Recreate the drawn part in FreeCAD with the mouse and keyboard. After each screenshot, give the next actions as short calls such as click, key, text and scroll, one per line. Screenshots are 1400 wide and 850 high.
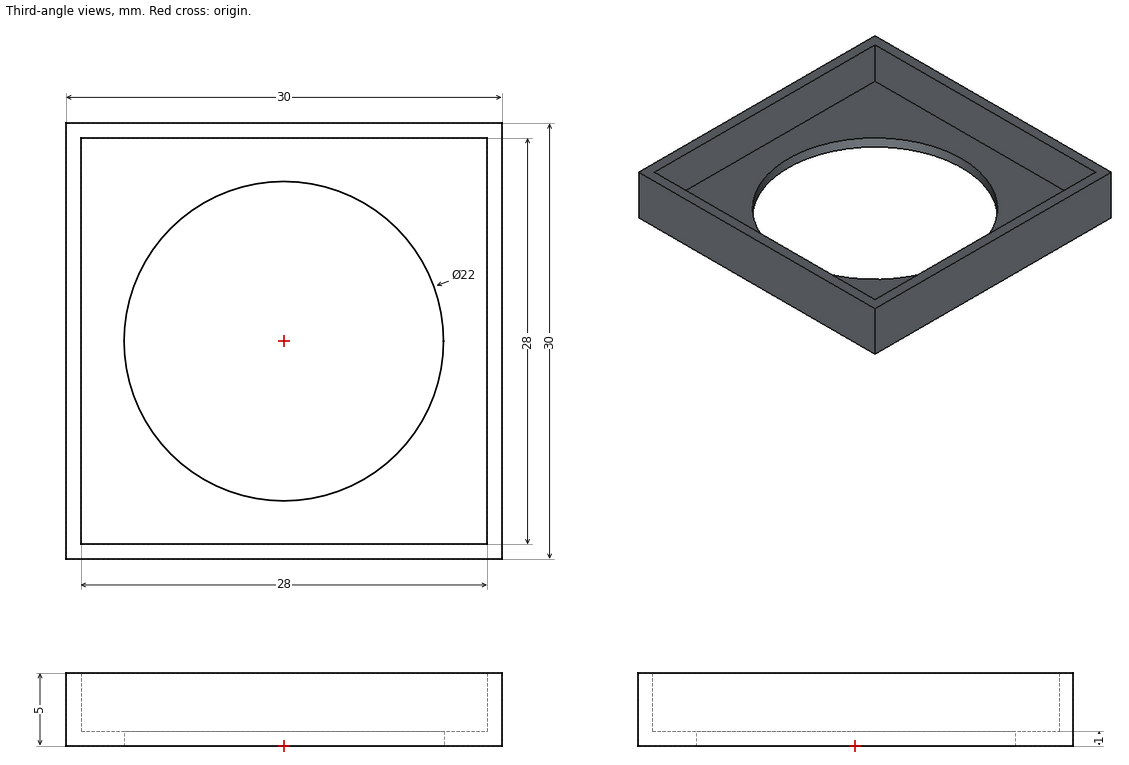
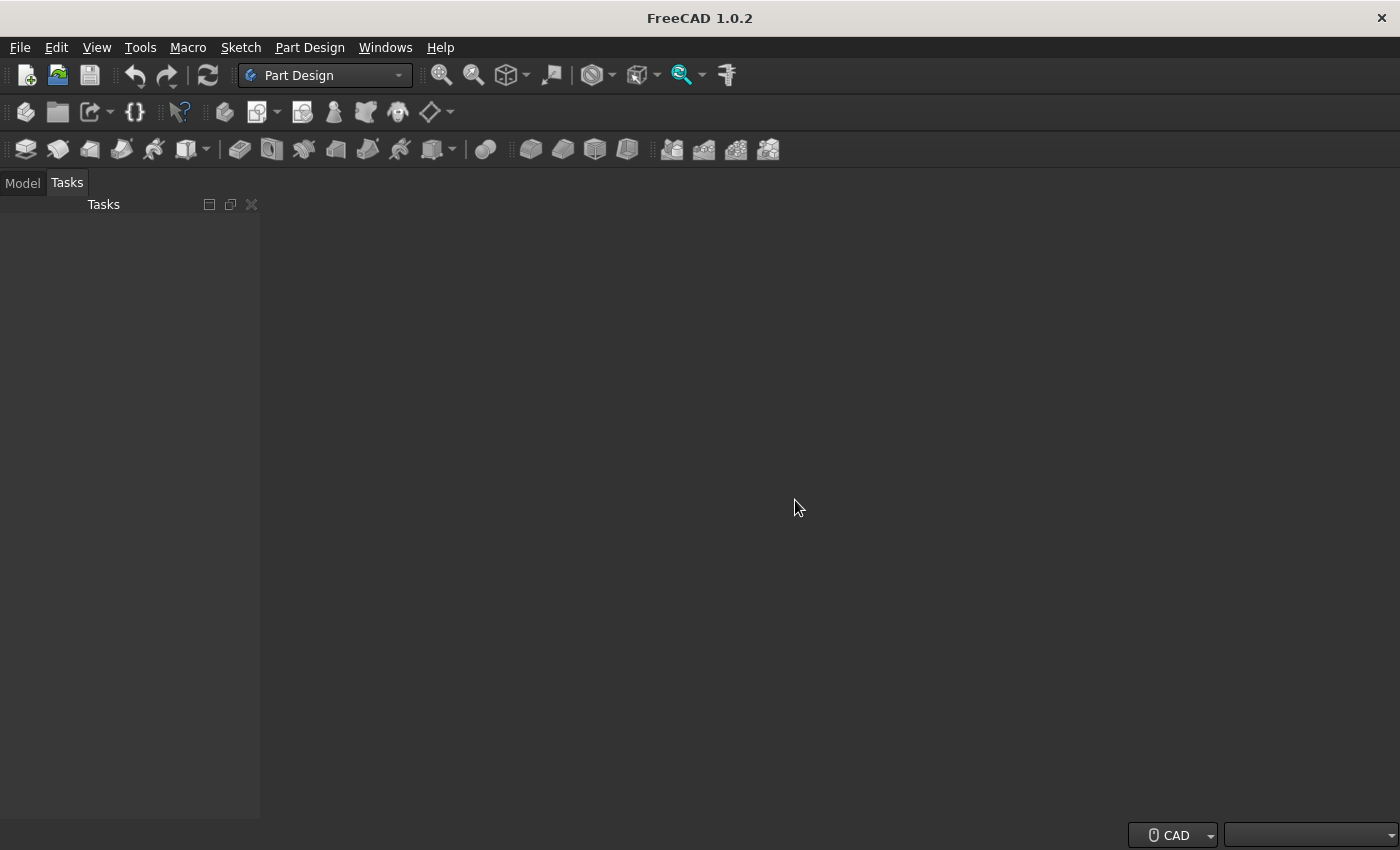
click(26, 76)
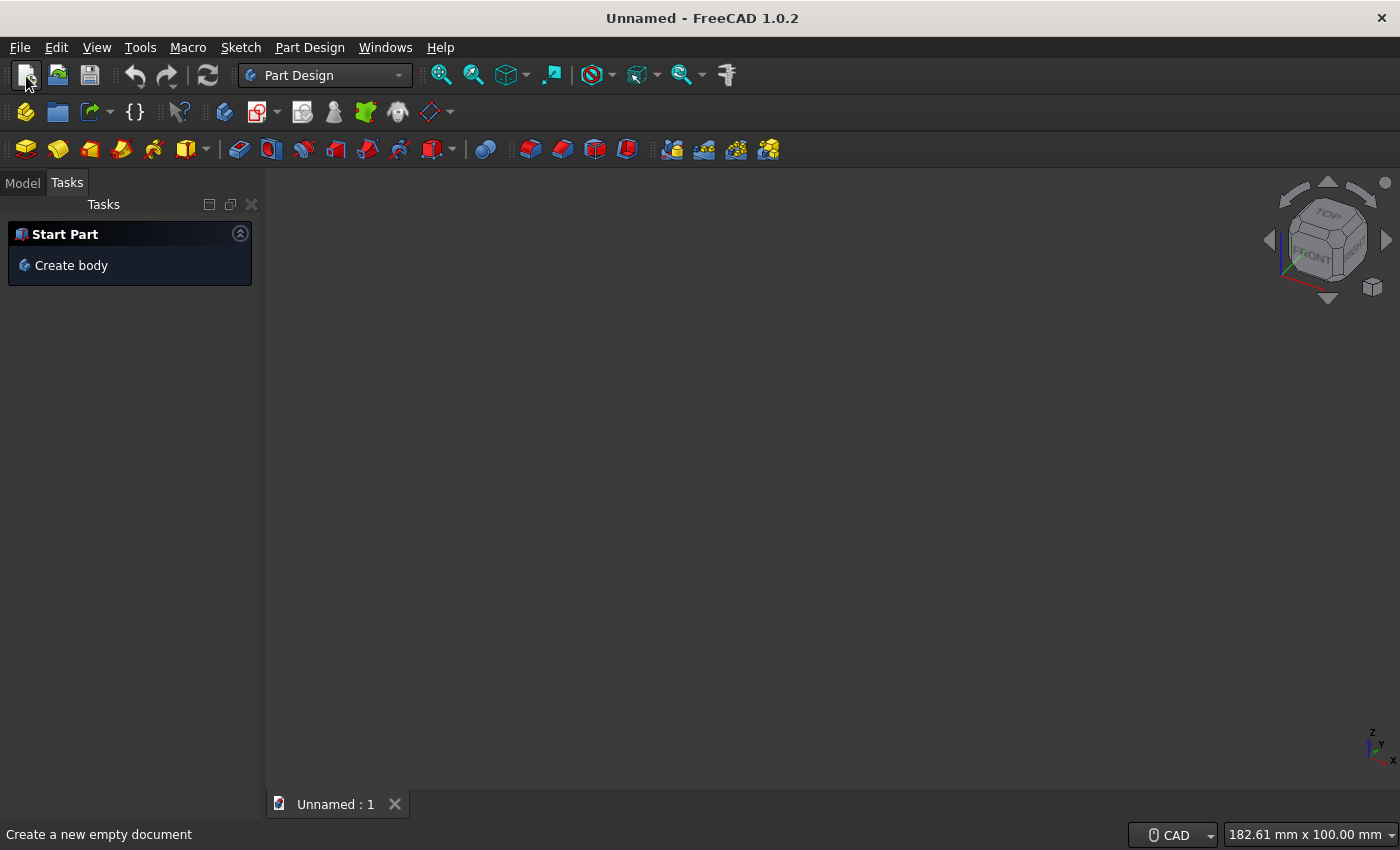
click(258, 112)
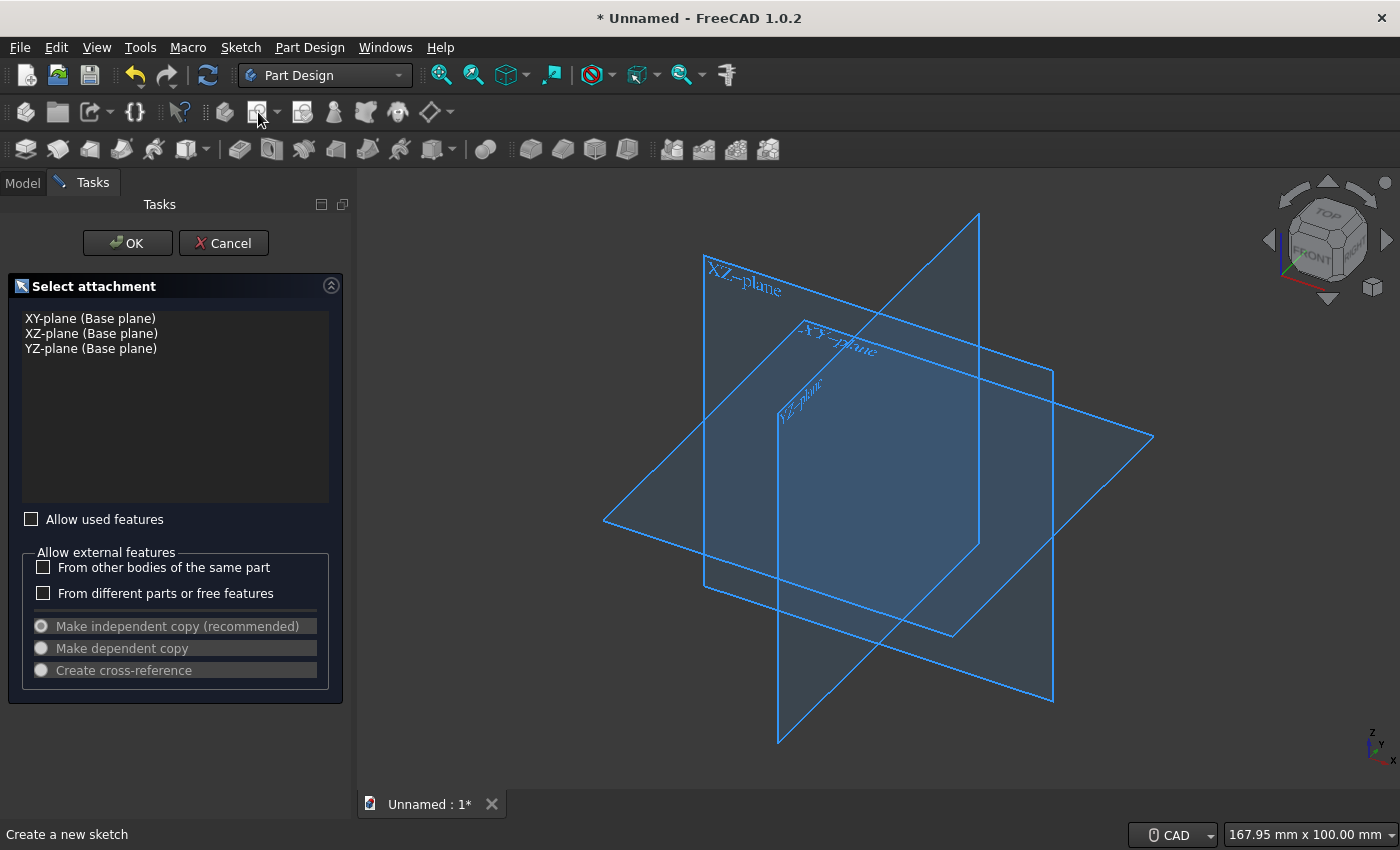
click(82, 318)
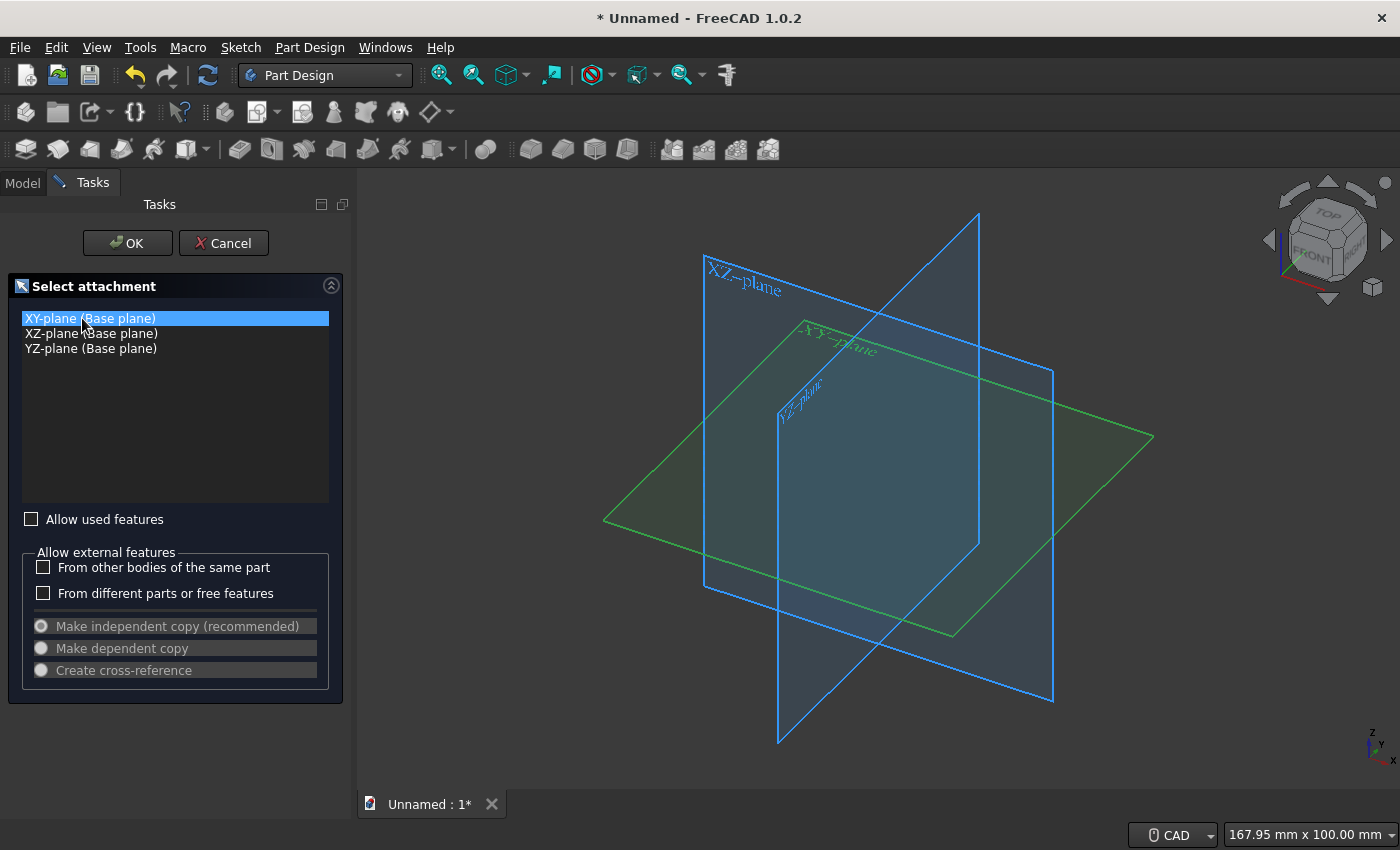
click(128, 243)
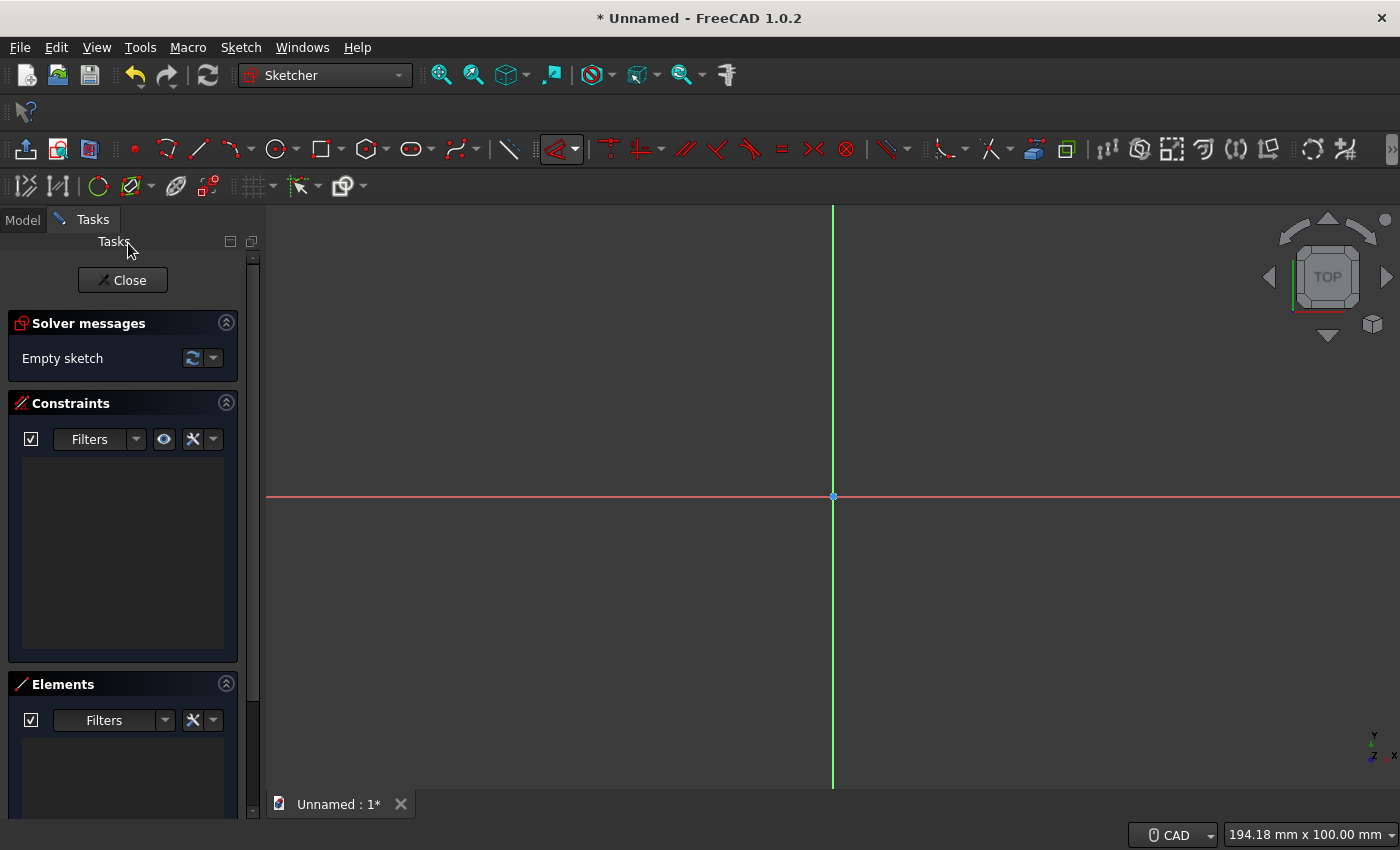
scroll(889, 497, up, 4)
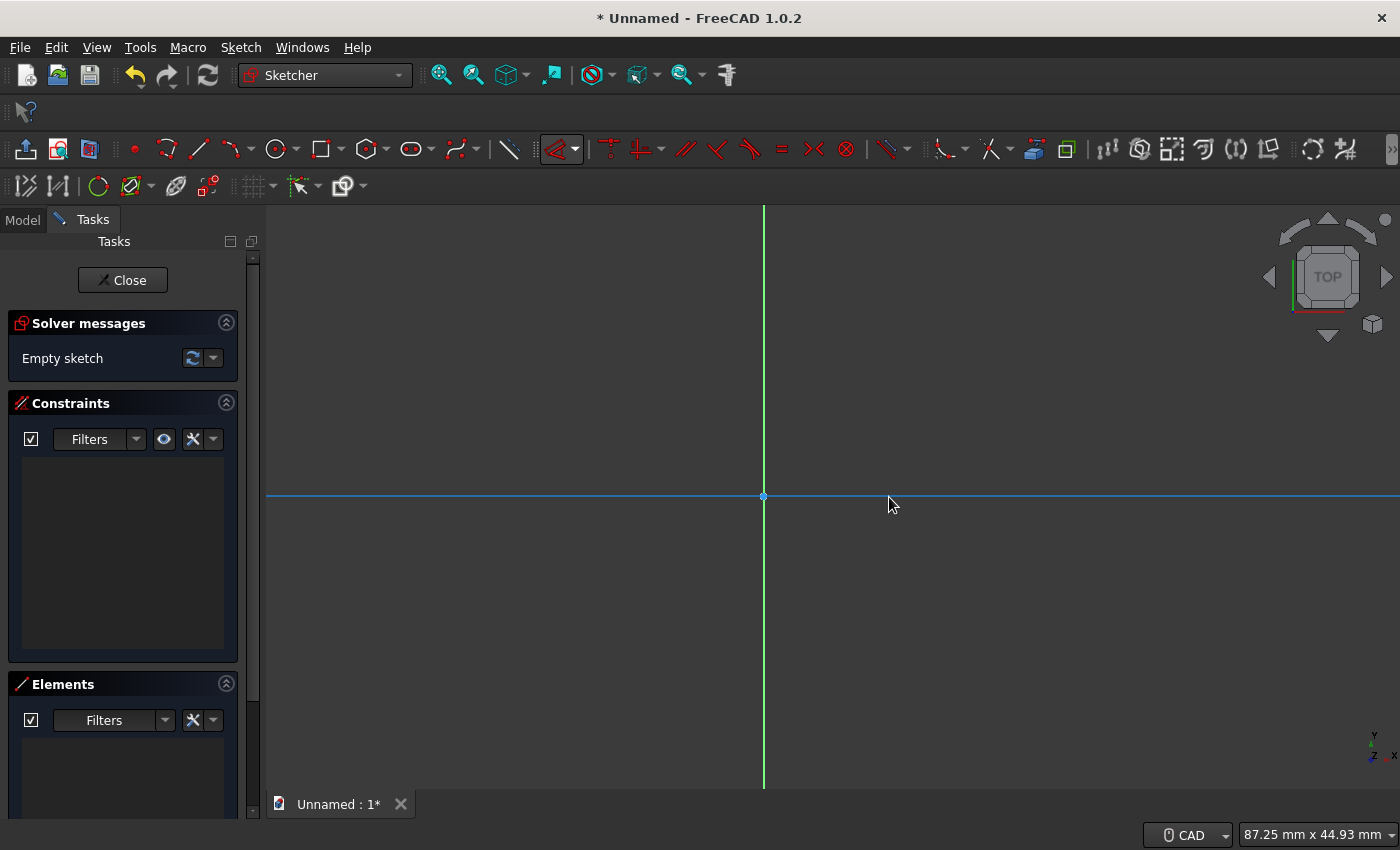
click(344, 150)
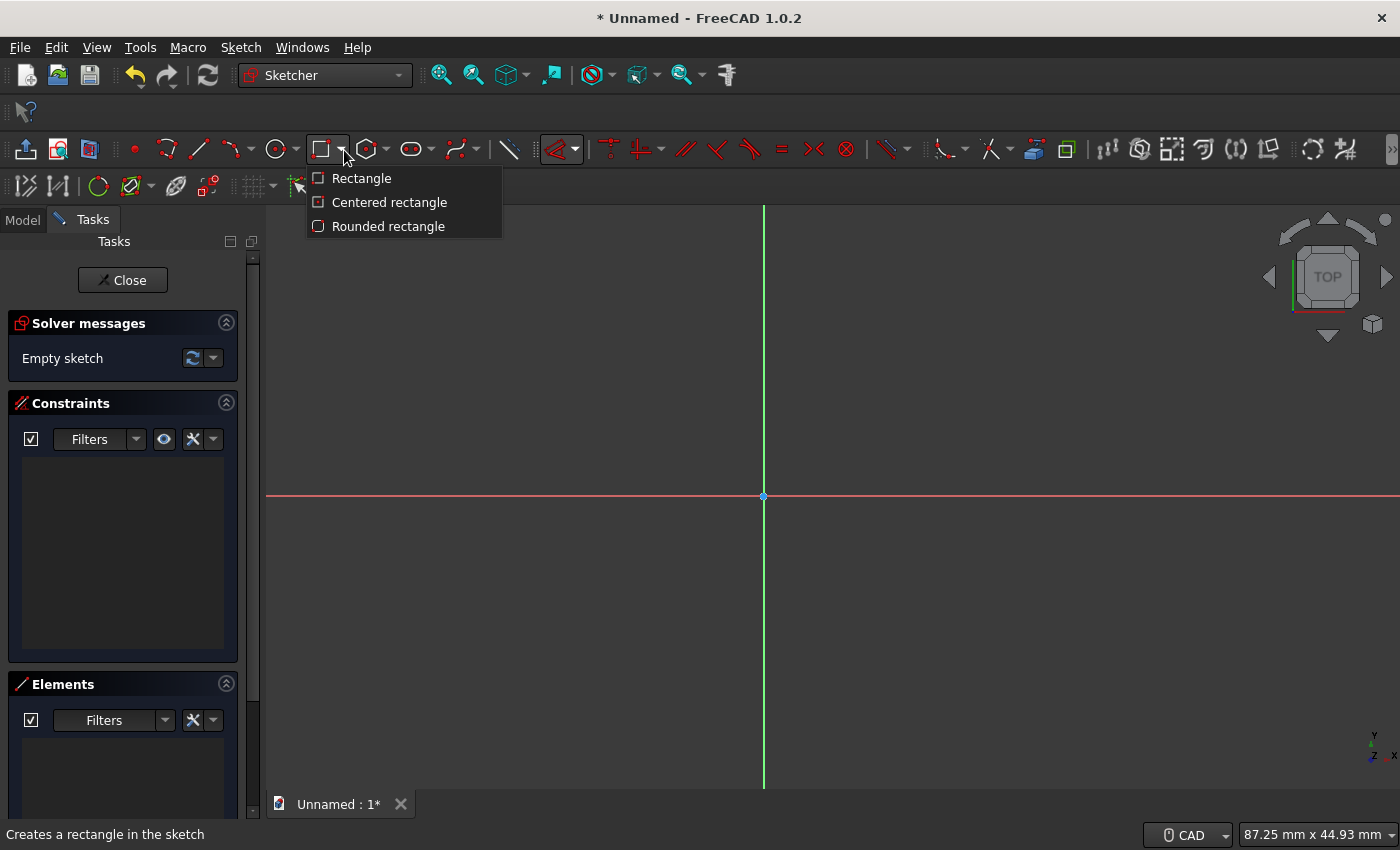
click(404, 202)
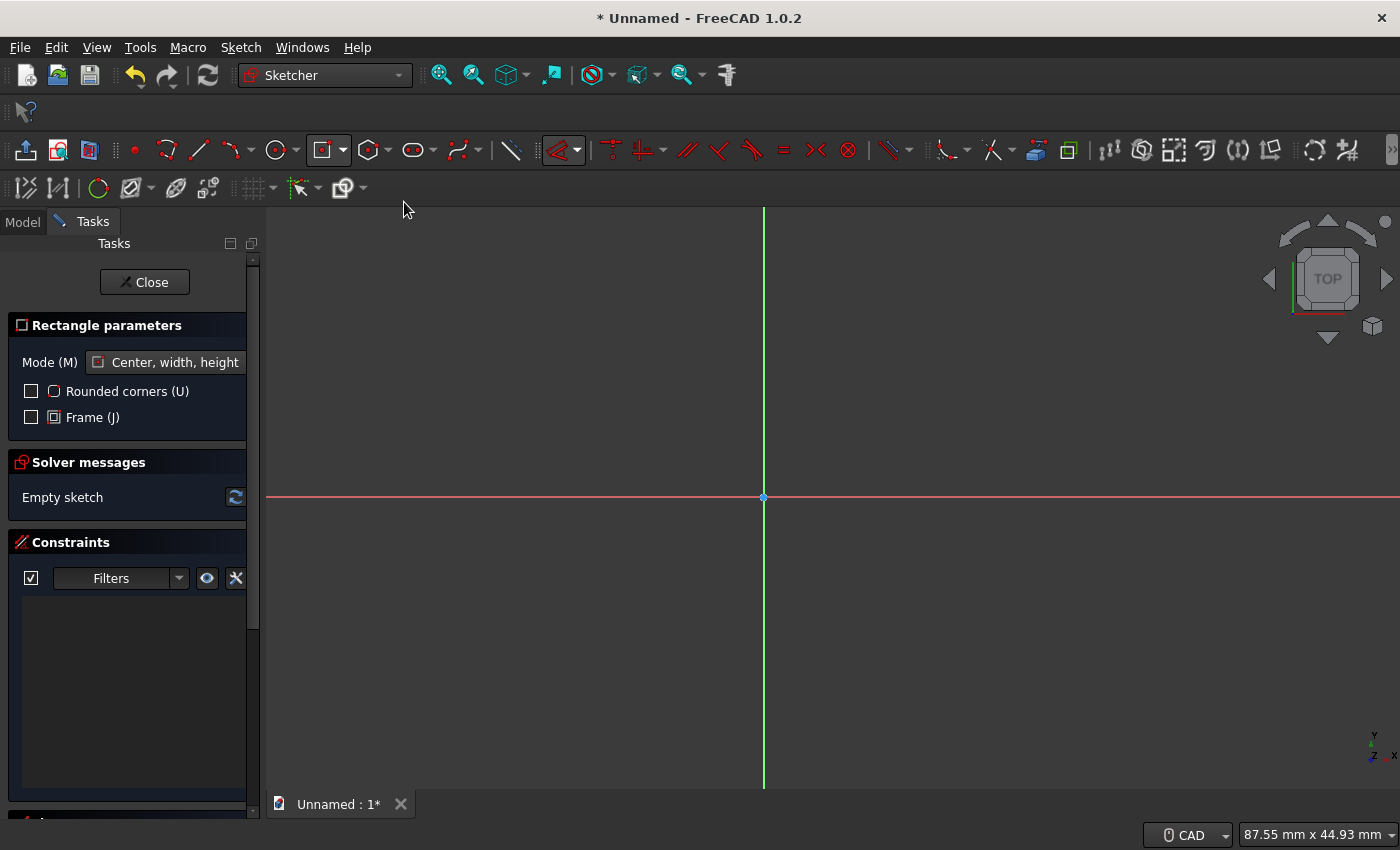
click(764, 497)
click(945, 316)
key(Escape)